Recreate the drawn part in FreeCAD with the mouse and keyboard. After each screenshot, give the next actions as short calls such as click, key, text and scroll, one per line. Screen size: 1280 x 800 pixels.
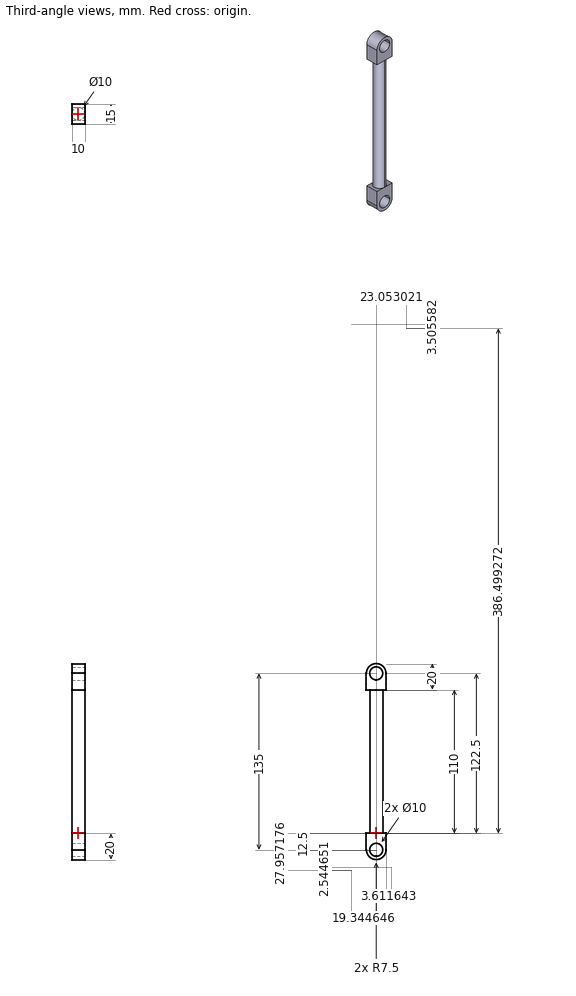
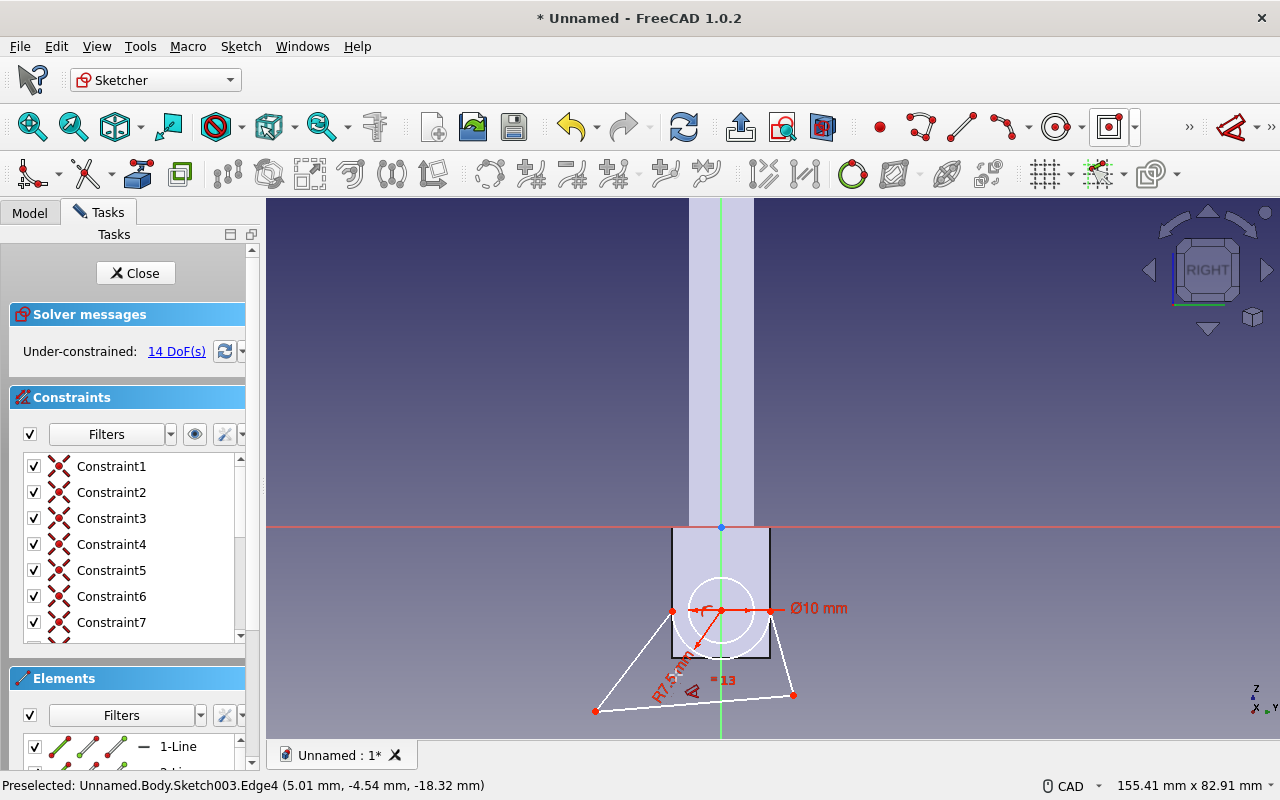
click(721, 610)
click(687, 569)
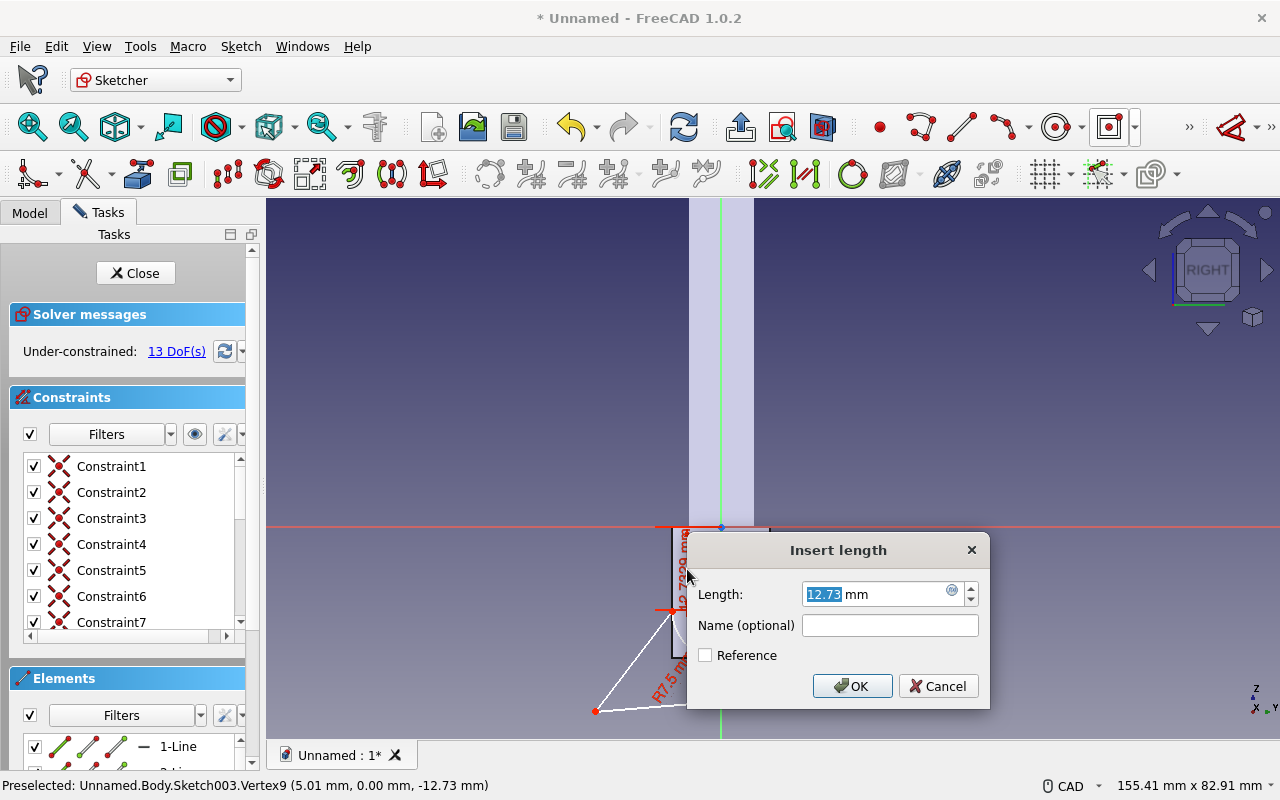
text(12.5)
key(Return)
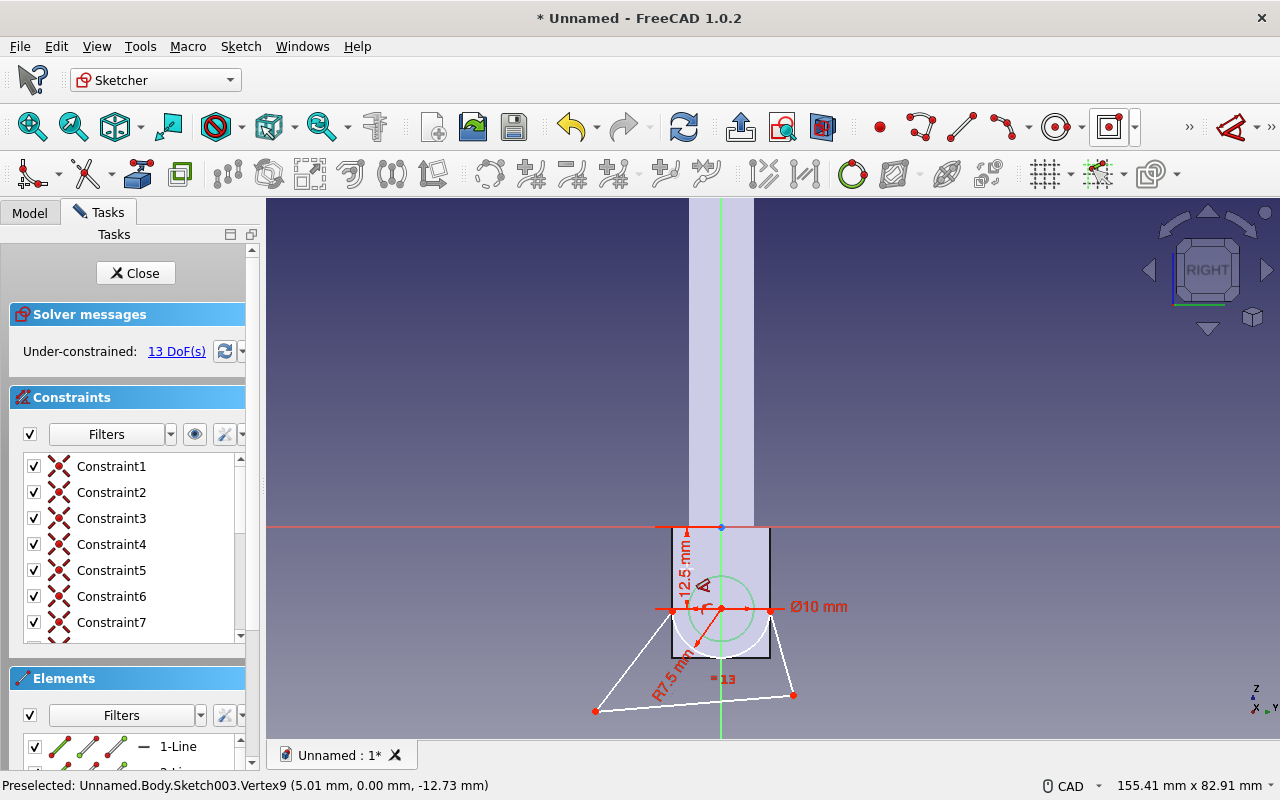
scroll(700, 644, down, 10)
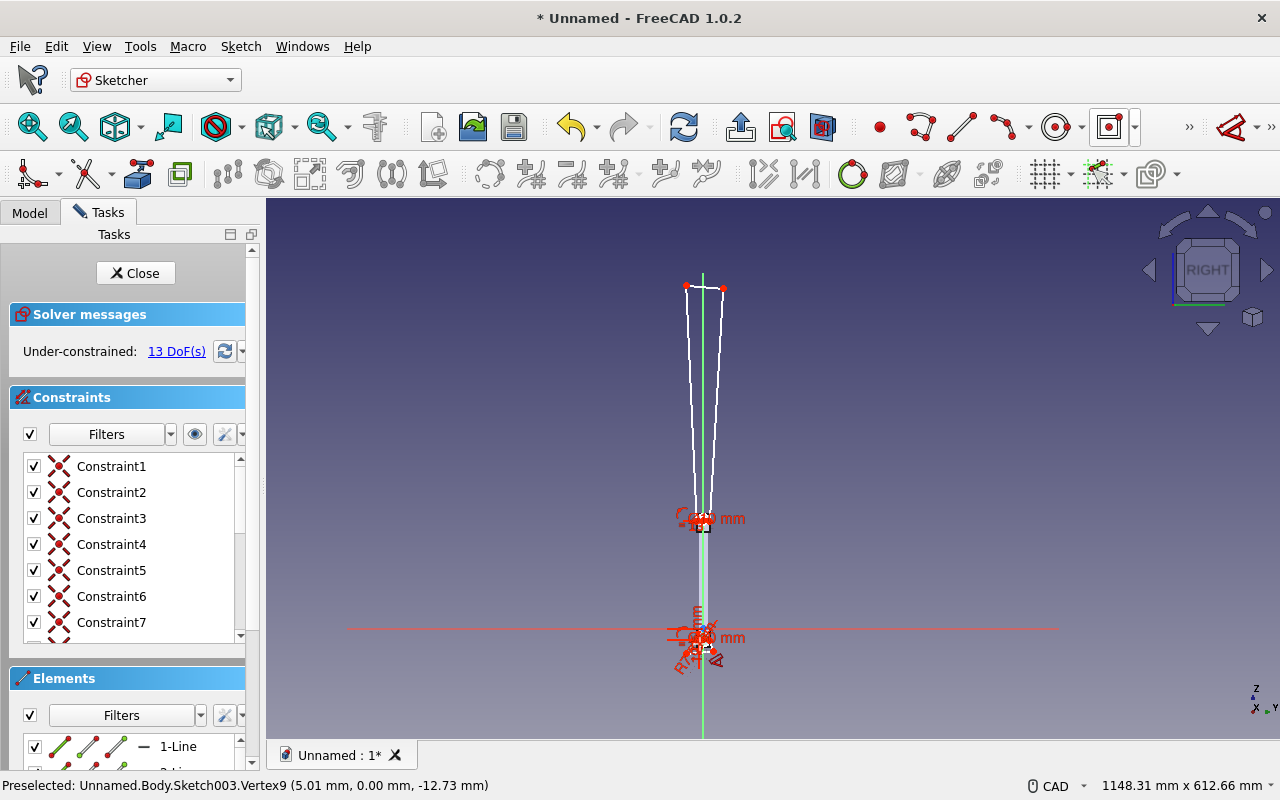
scroll(703, 640, up, 4)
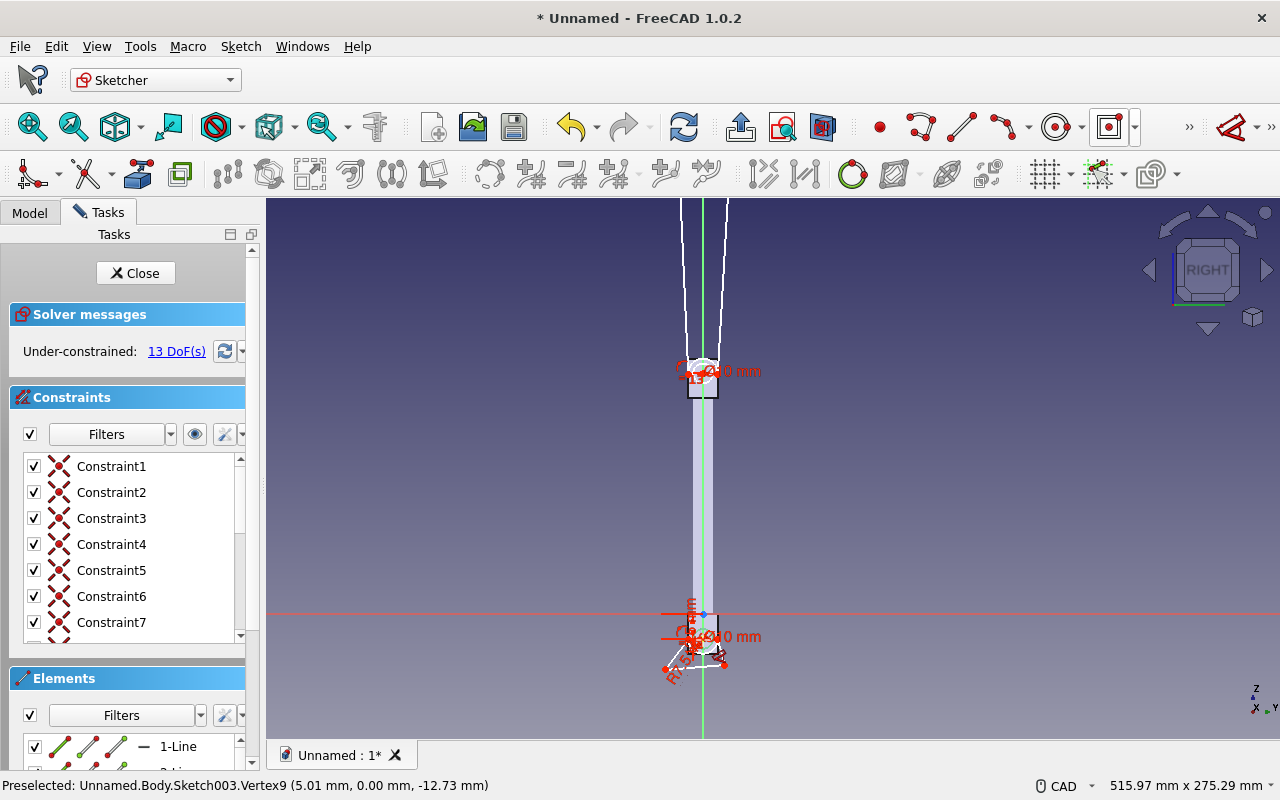
click(703, 639)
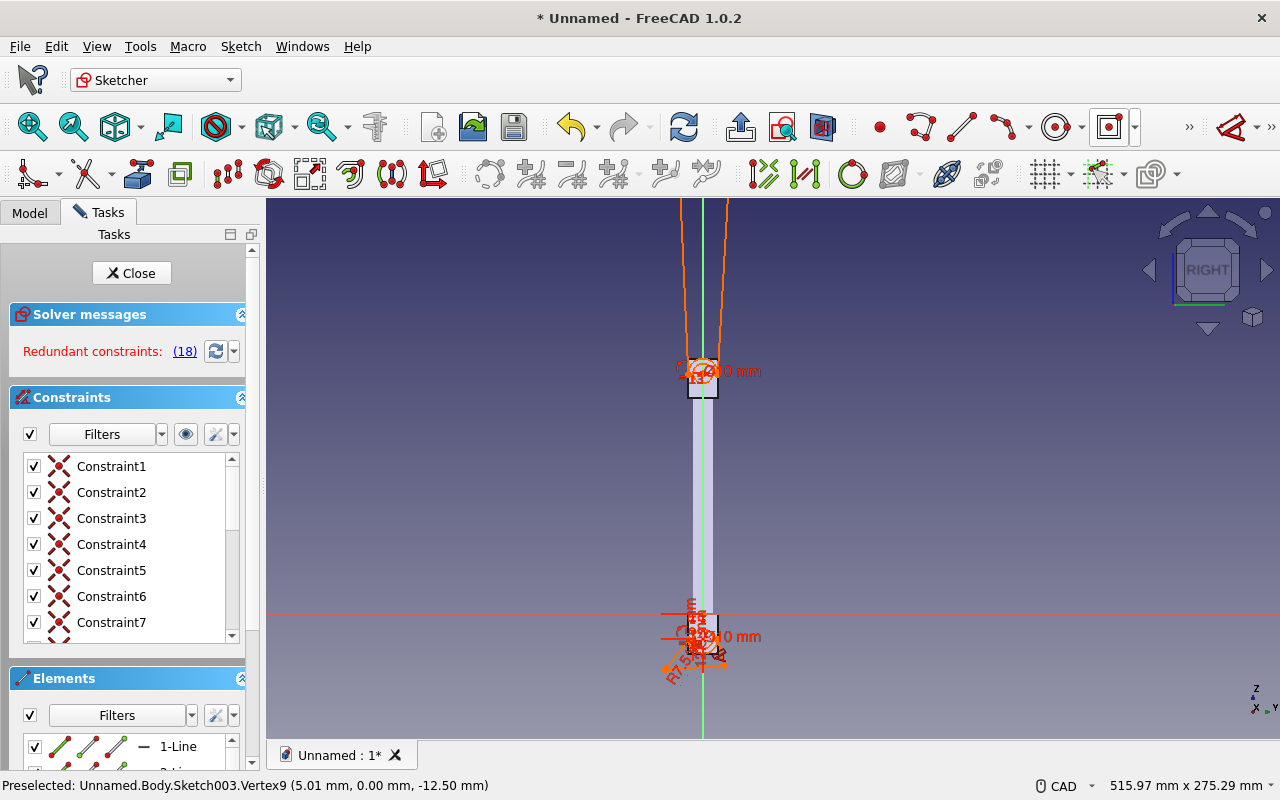
click(703, 373)
click(669, 506)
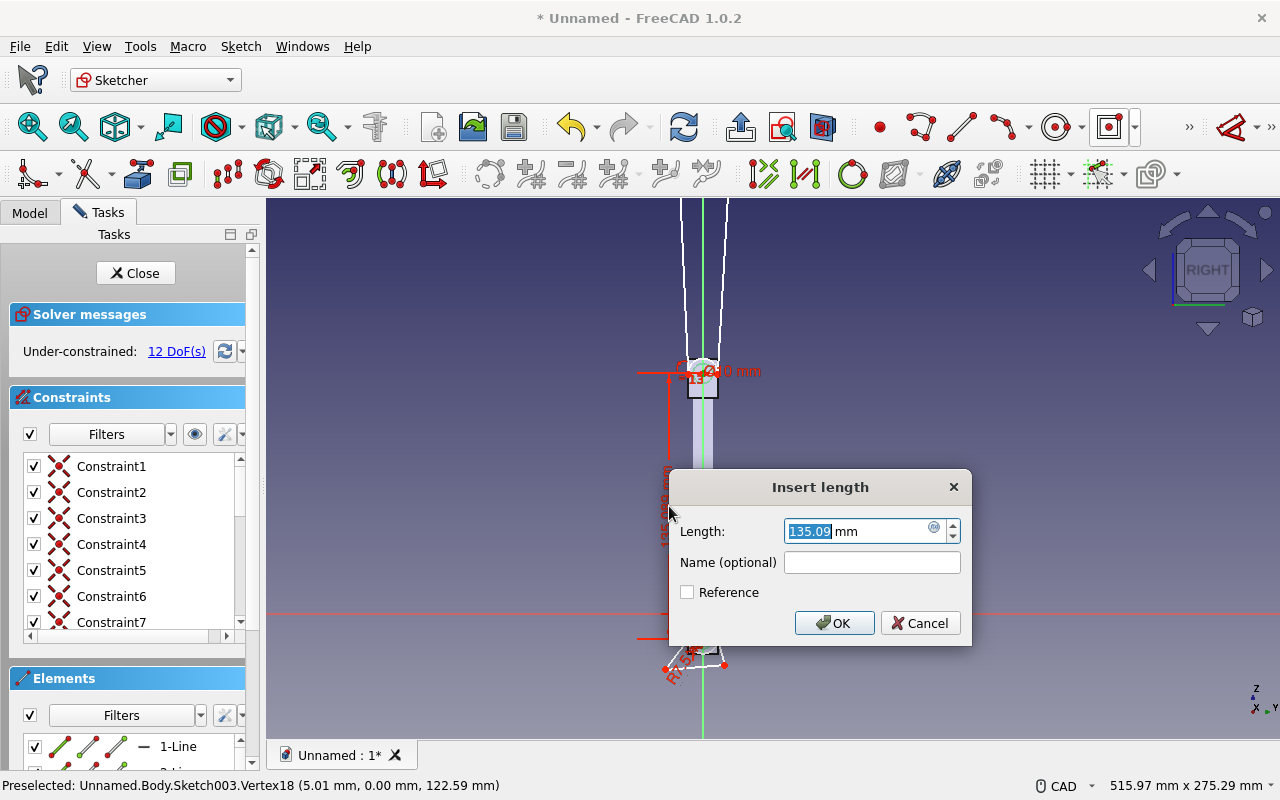
text(135)
key(Return)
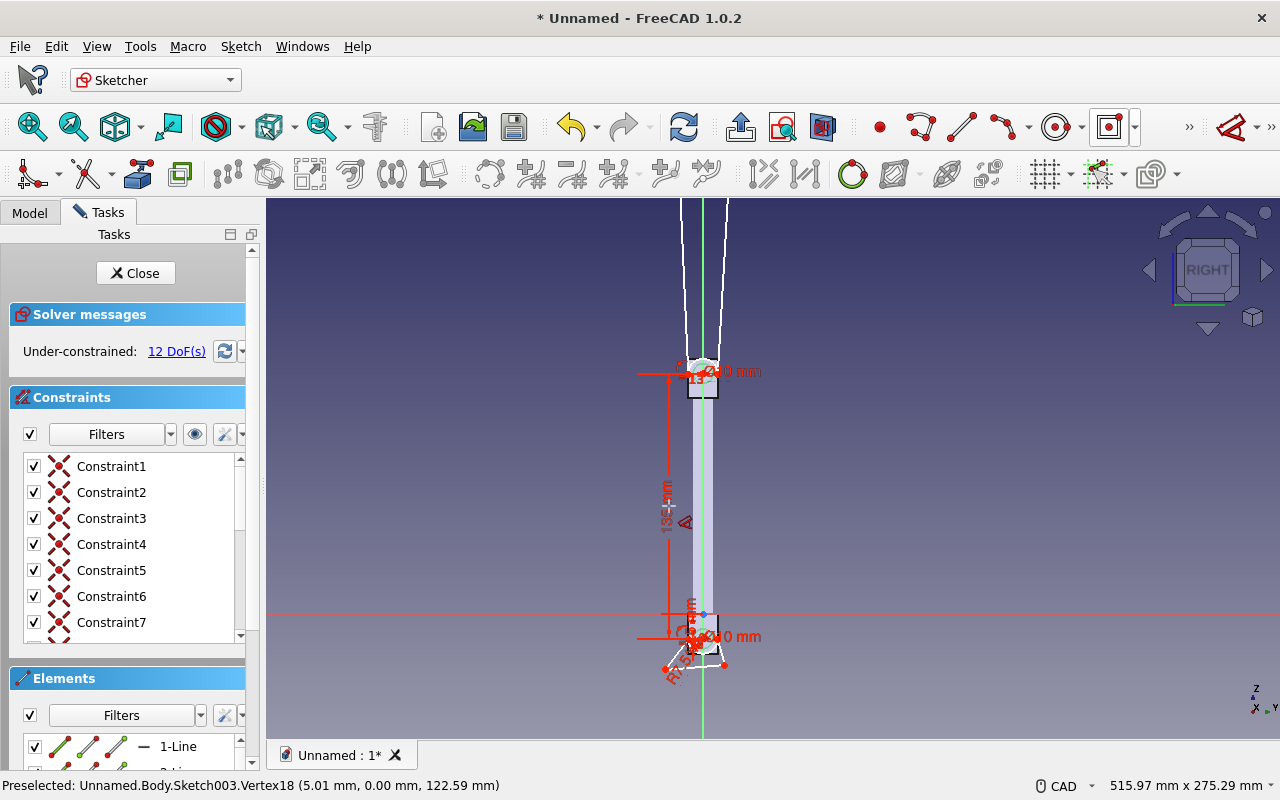
click(688, 640)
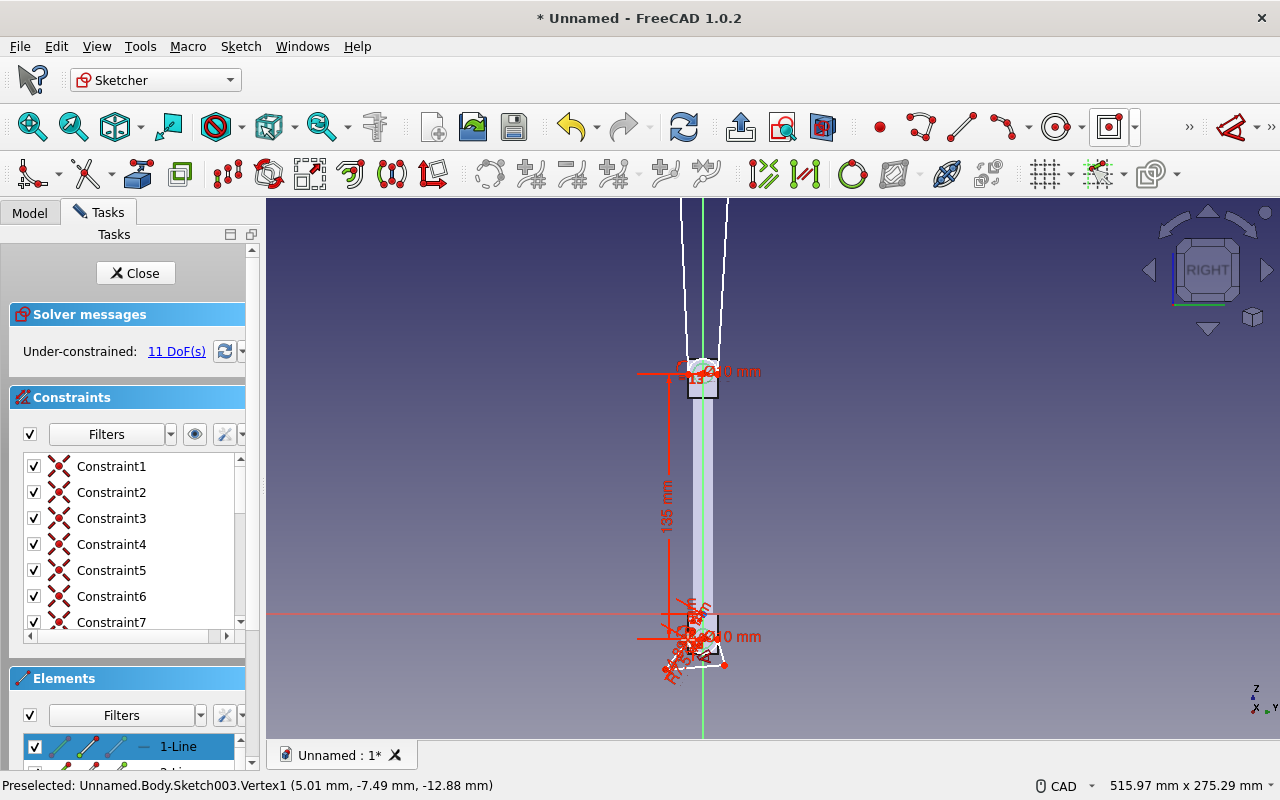
click(703, 374)
click(654, 445)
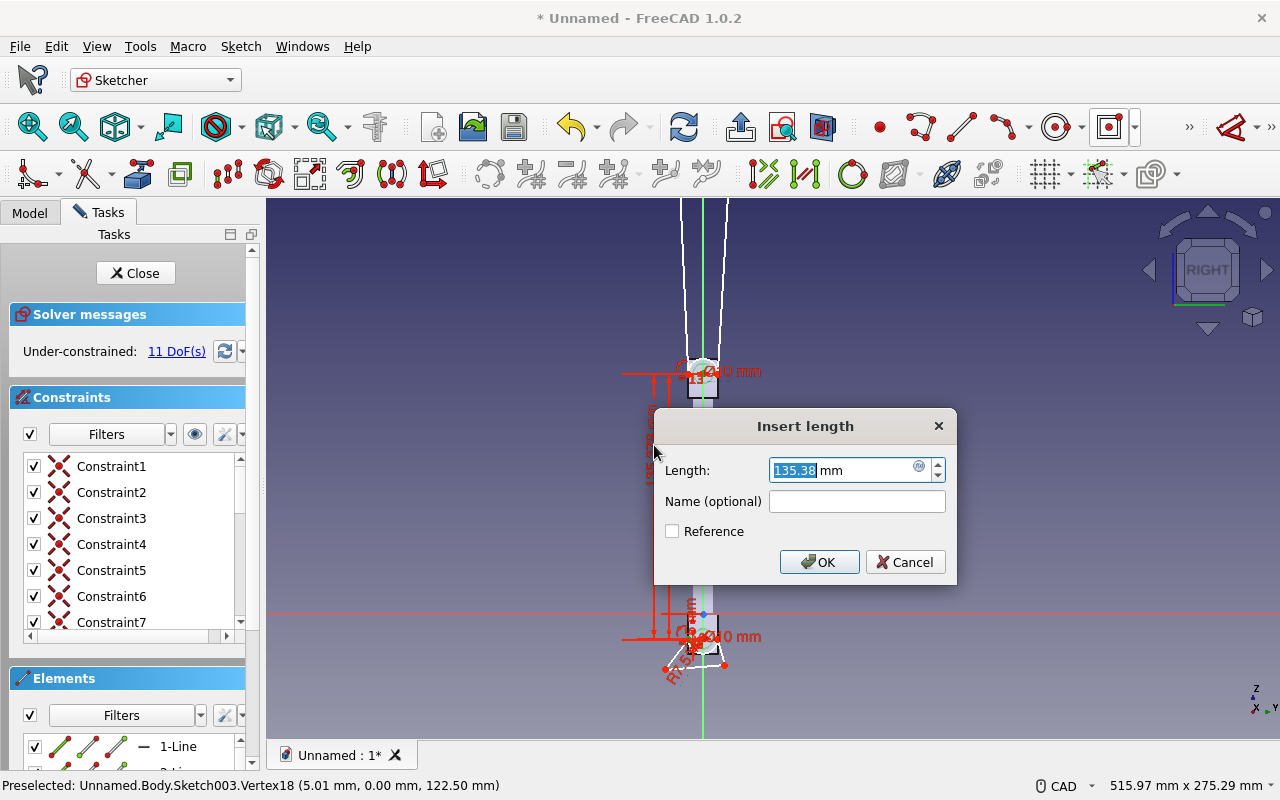
text(135)
key(Return)